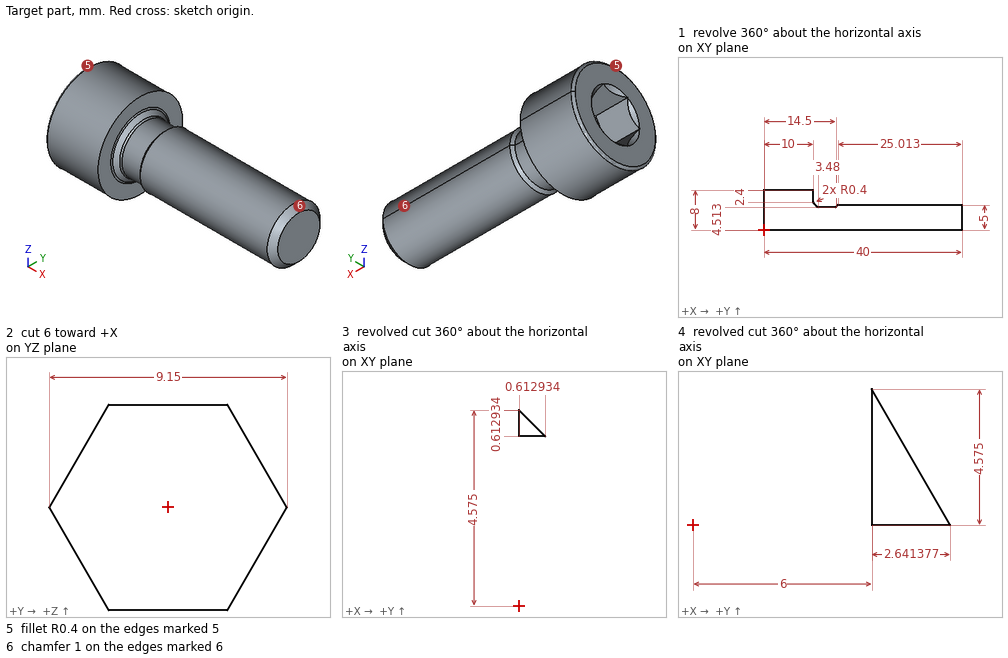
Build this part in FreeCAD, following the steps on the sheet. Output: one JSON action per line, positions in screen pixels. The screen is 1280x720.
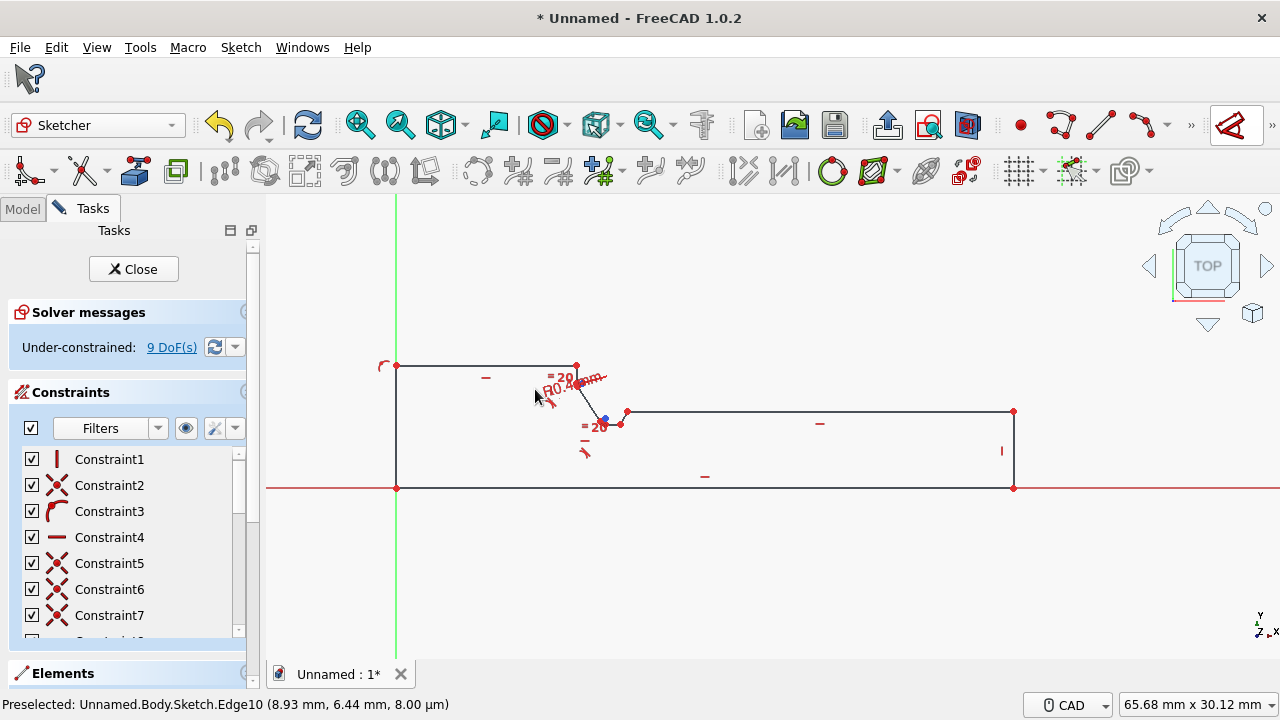
{"action": "left_click", "coordinate": [396, 403]}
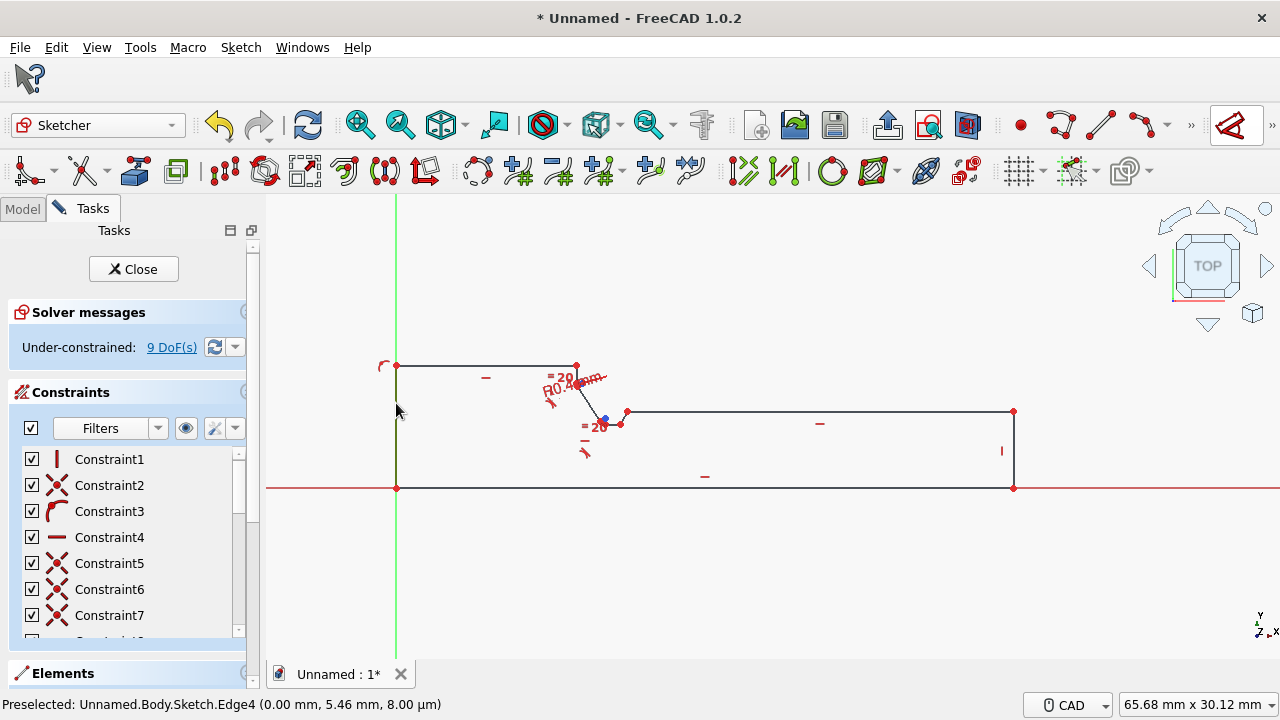
{"action": "left_click", "coordinate": [1258, 126]}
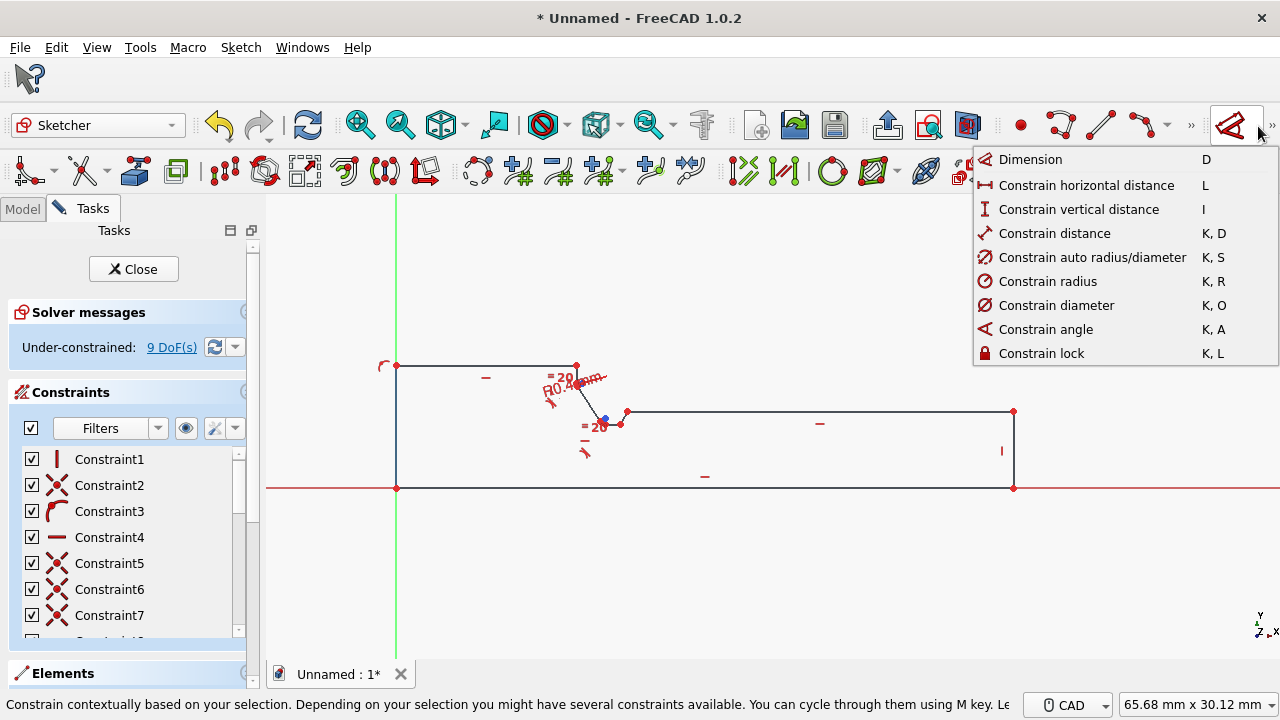
{"action": "left_click", "coordinate": [1126, 209]}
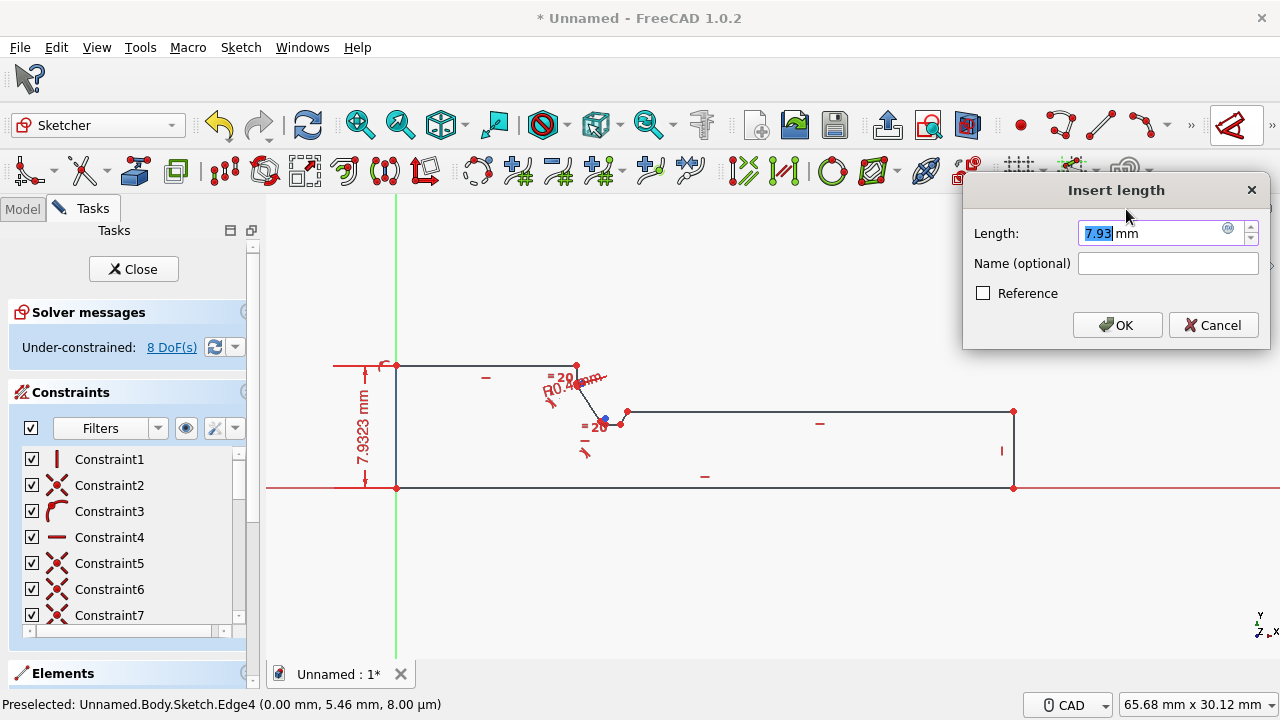
{"action": "type", "text": "8"}
{"action": "key", "text": "Return"}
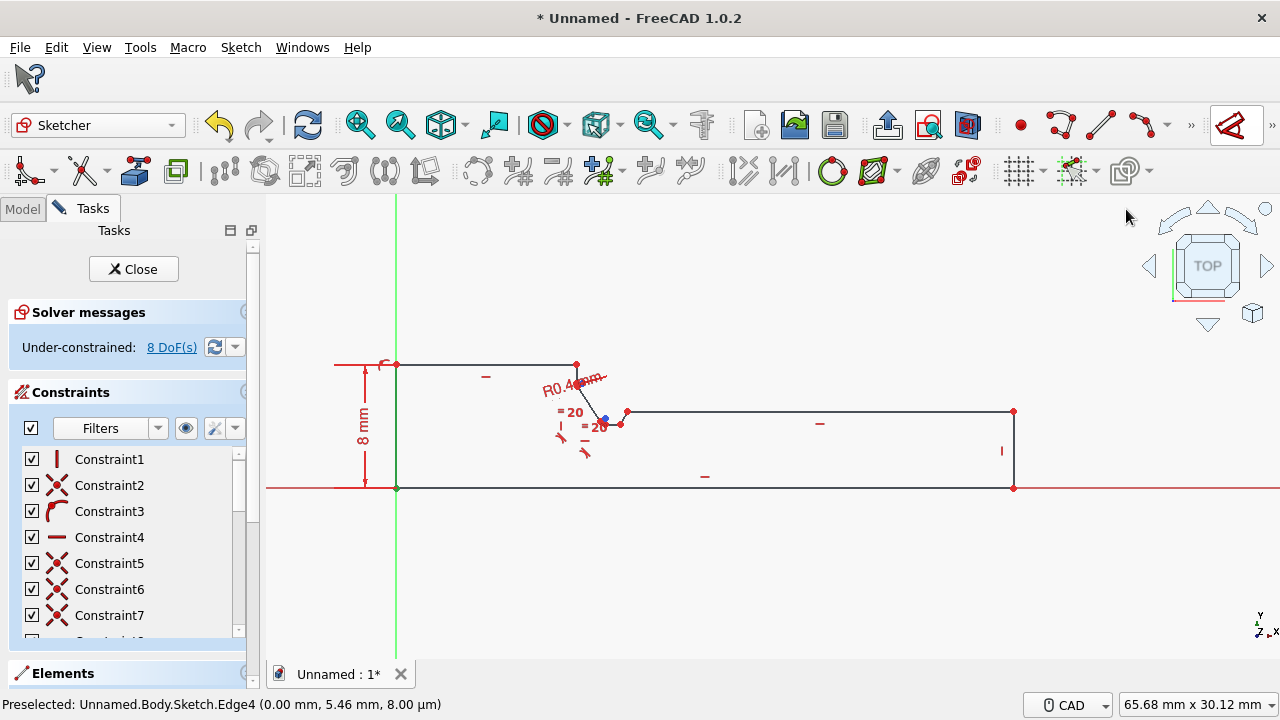
{"action": "left_click", "coordinate": [1014, 465]}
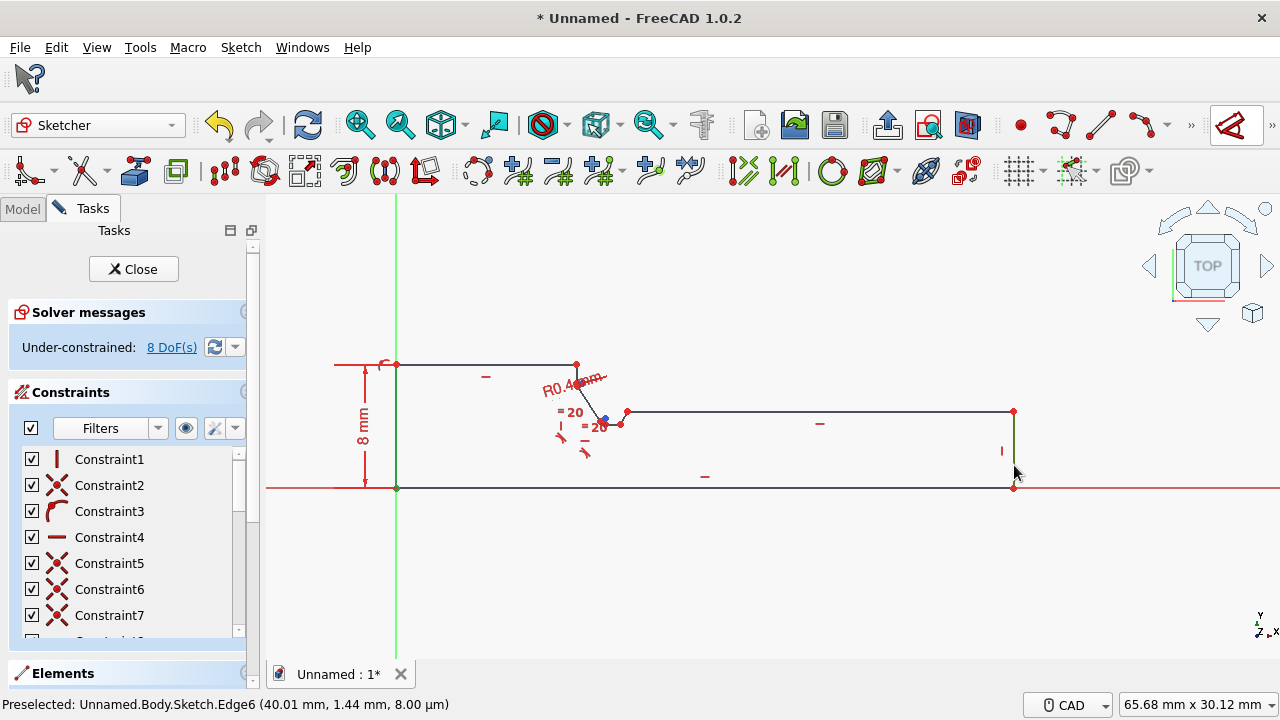
{"action": "left_click", "coordinate": [1258, 126]}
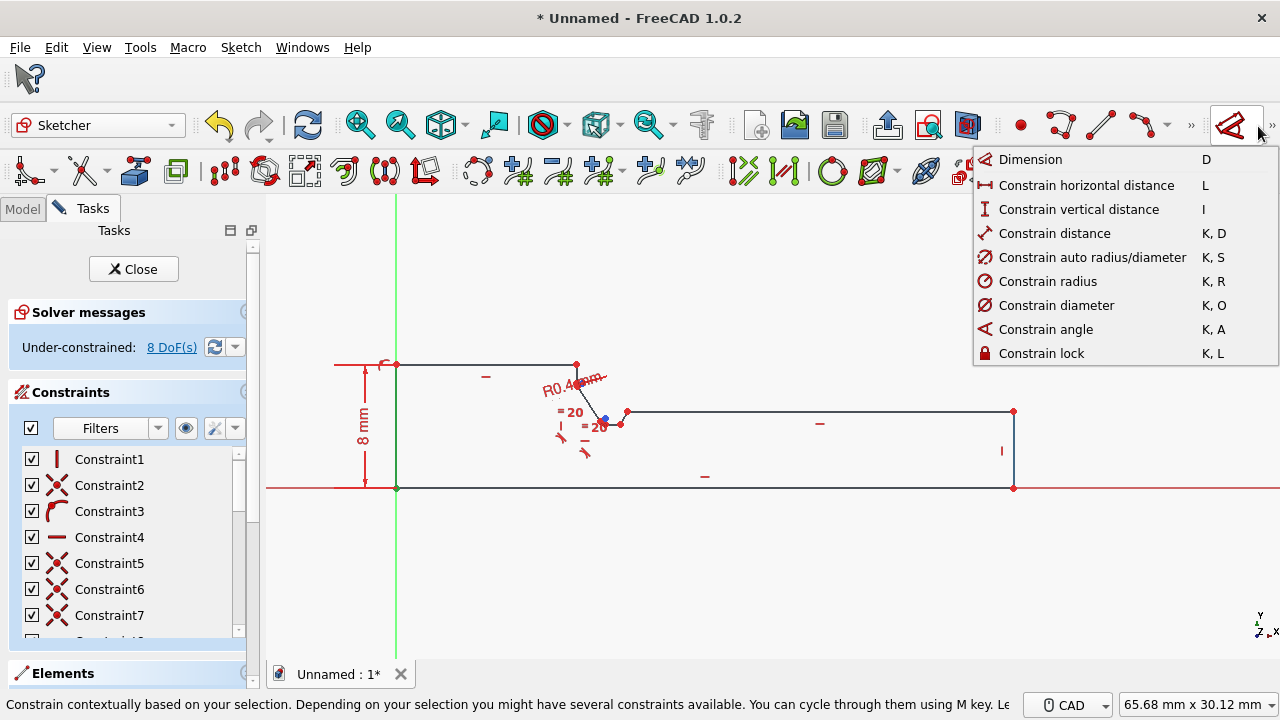
{"action": "left_click", "coordinate": [1126, 209]}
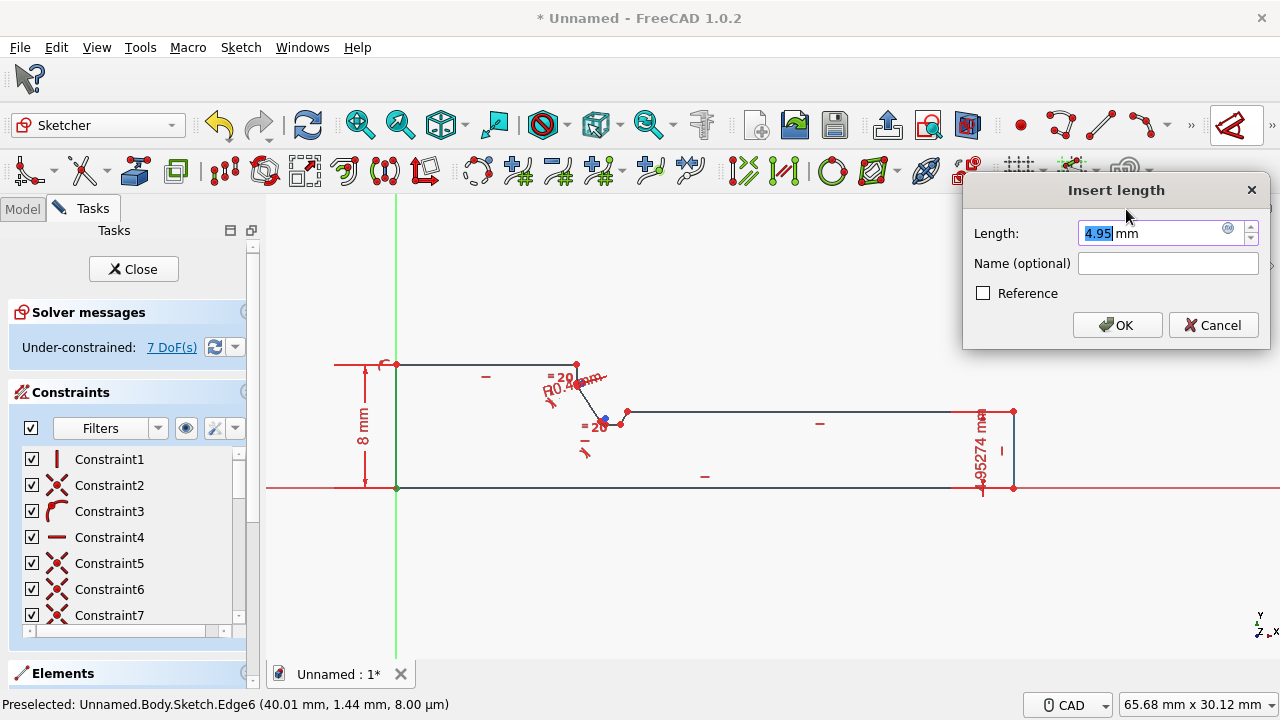
{"action": "type", "text": "5"}
{"action": "key", "text": "Return"}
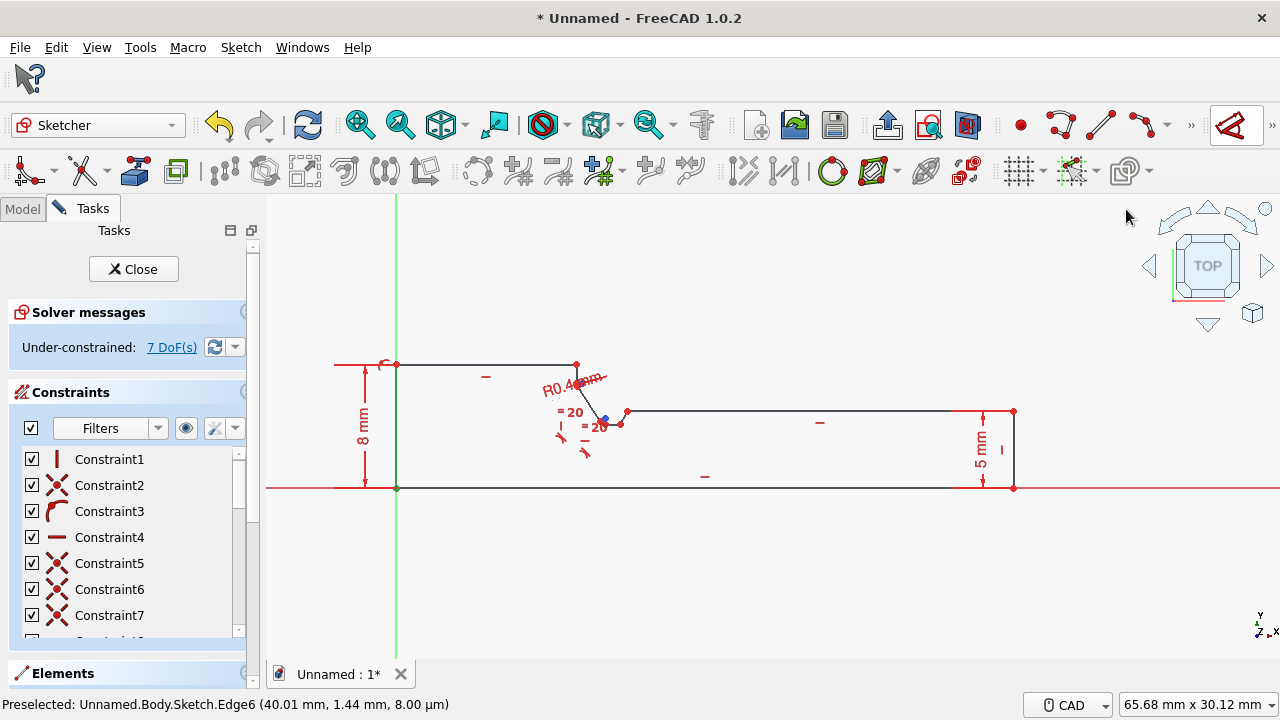
{"action": "left_click", "coordinate": [523, 365]}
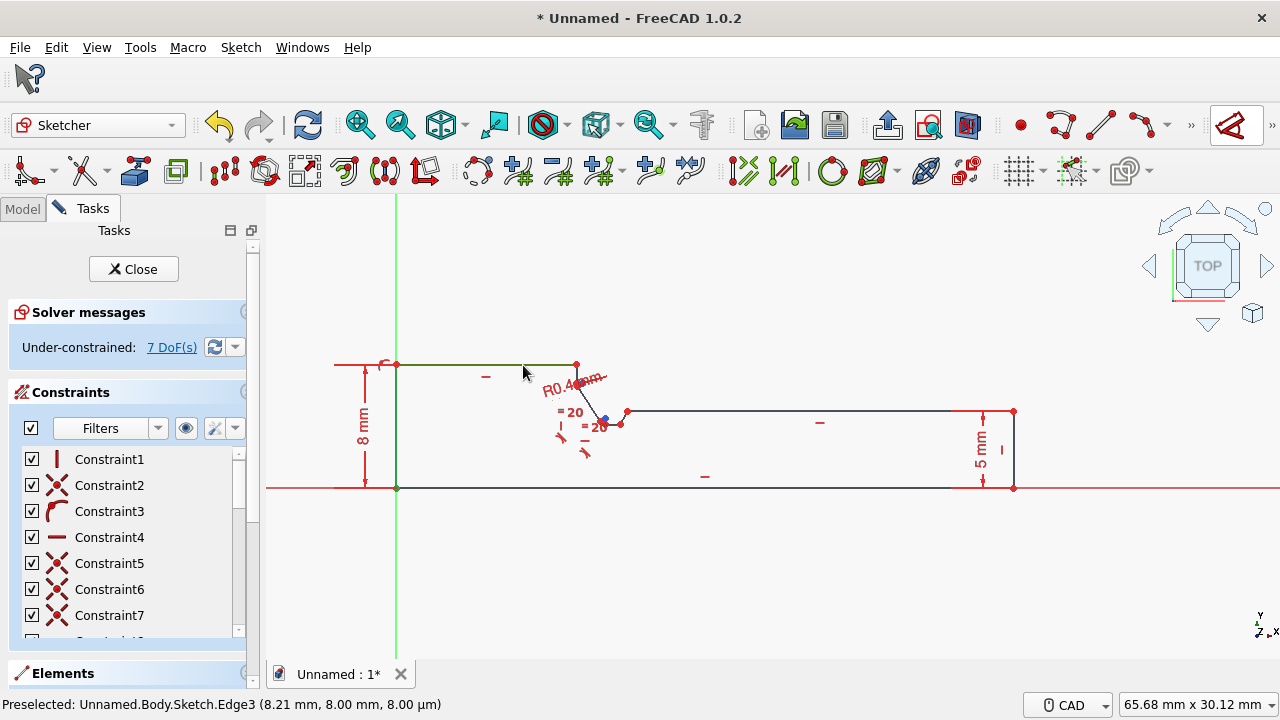
{"action": "key", "text": "l"}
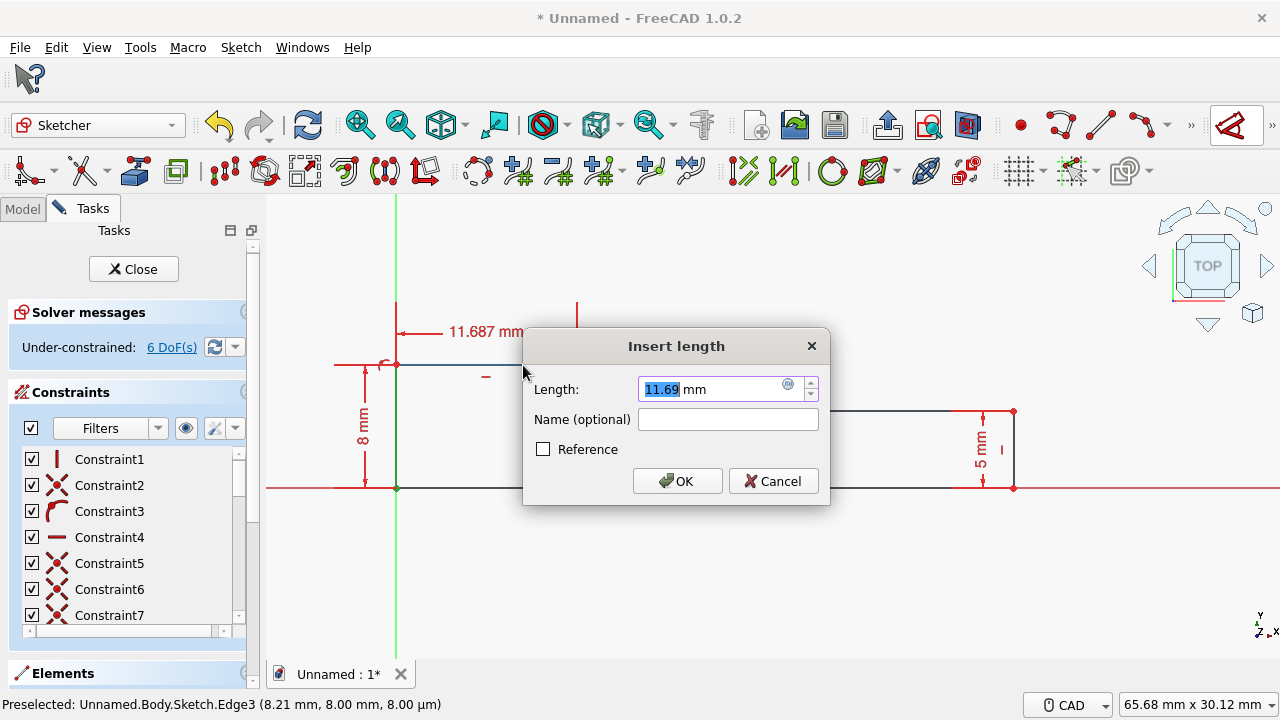
{"action": "type", "text": "10"}
{"action": "key", "text": "Return"}